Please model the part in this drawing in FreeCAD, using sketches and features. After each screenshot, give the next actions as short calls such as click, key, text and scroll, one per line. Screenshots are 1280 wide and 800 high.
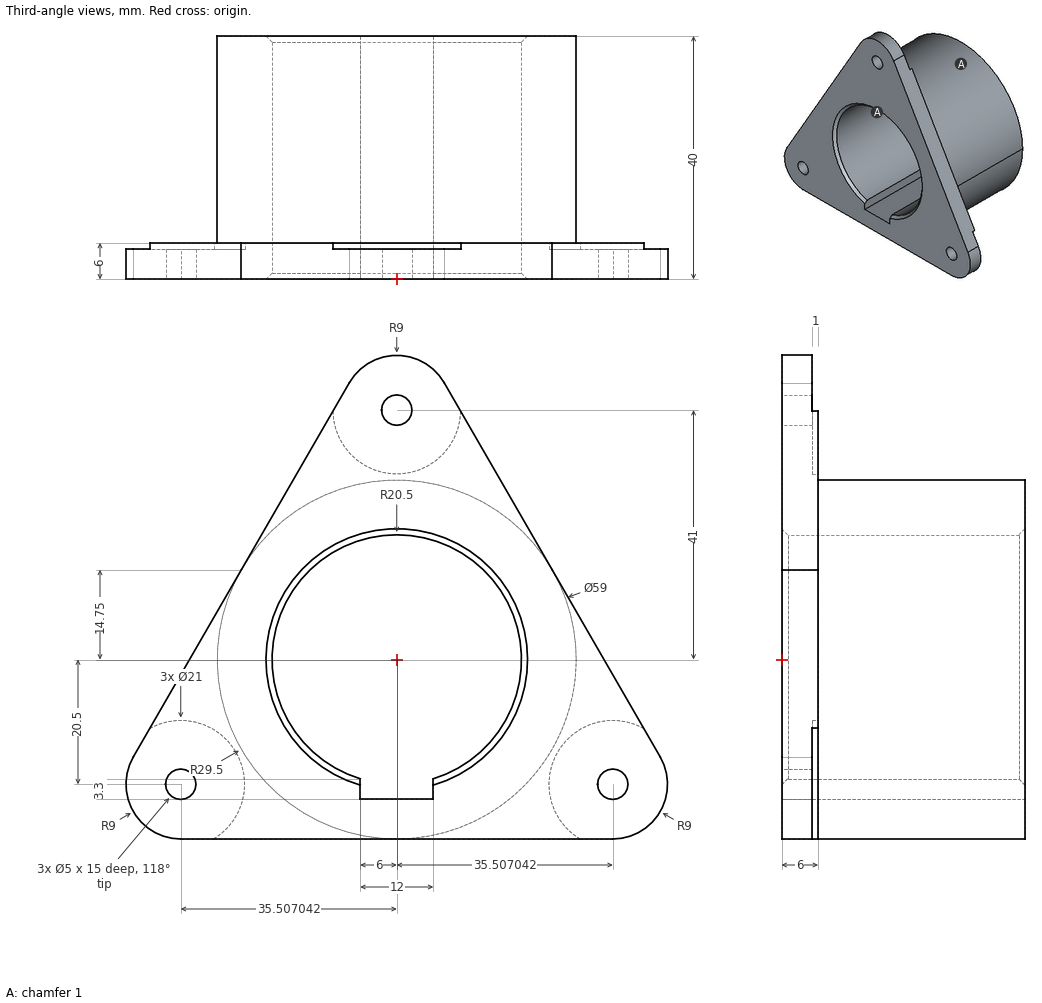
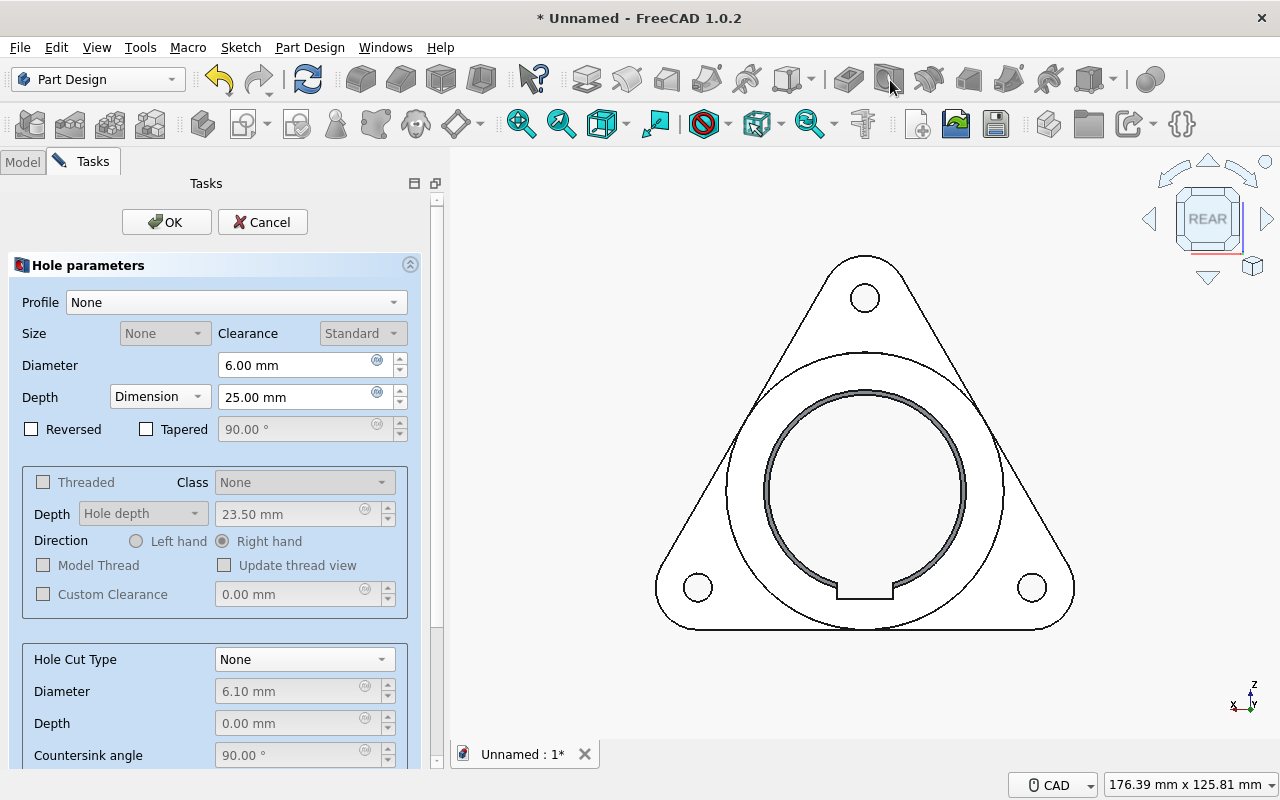
triple_click(305, 365)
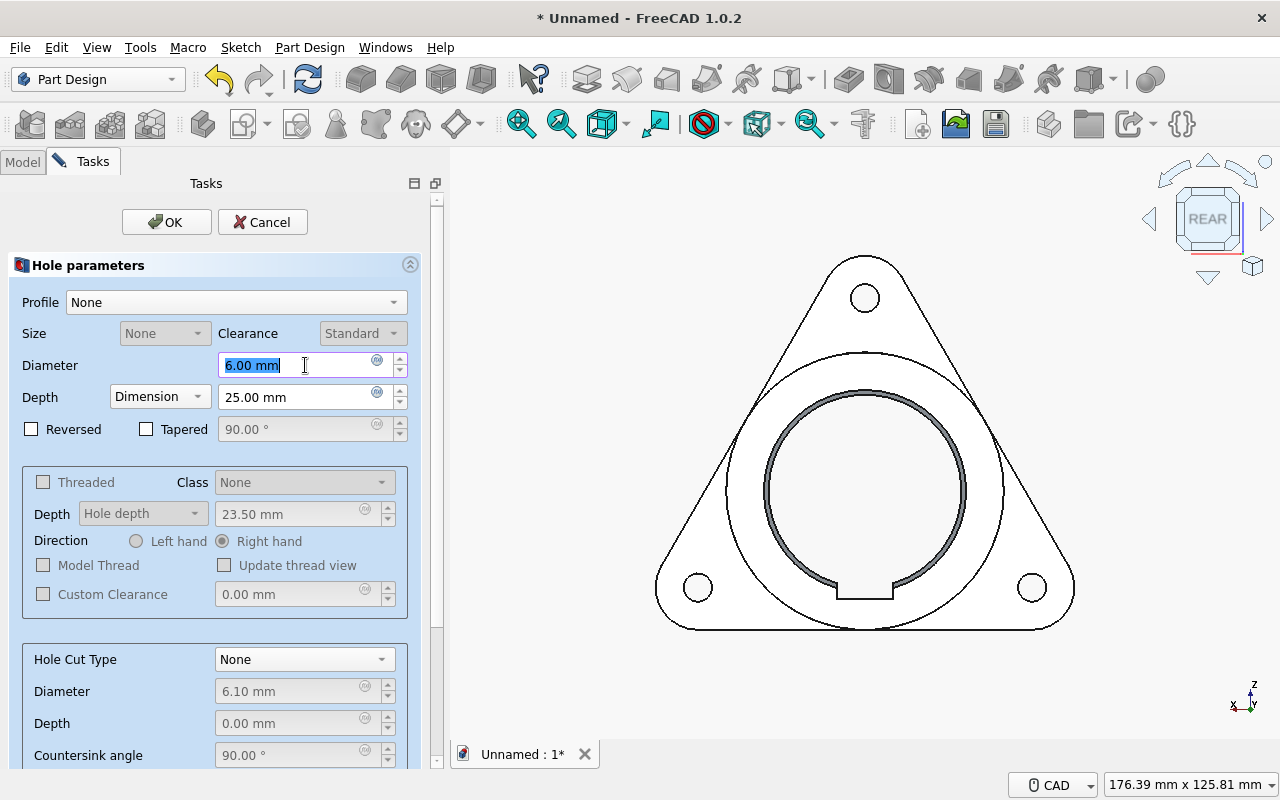
text(5)
key(Tab)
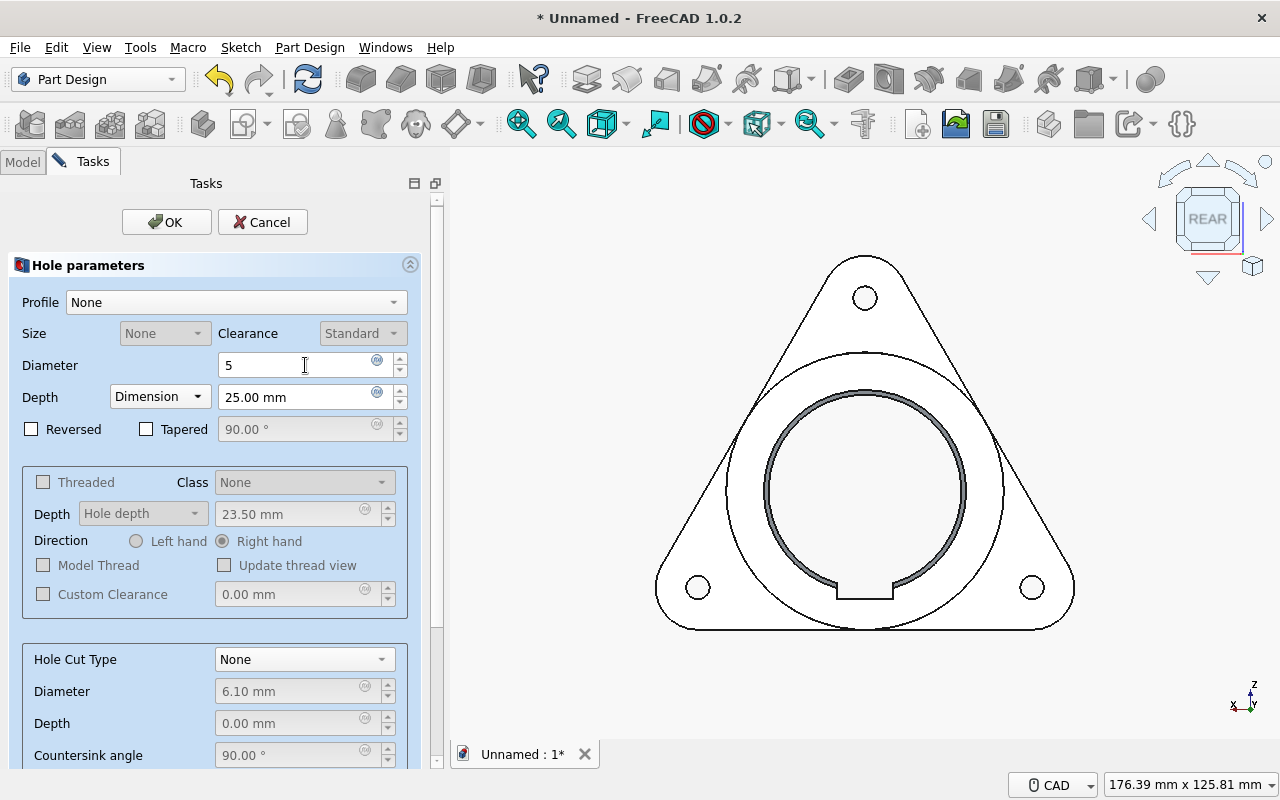
triple_click(305, 397)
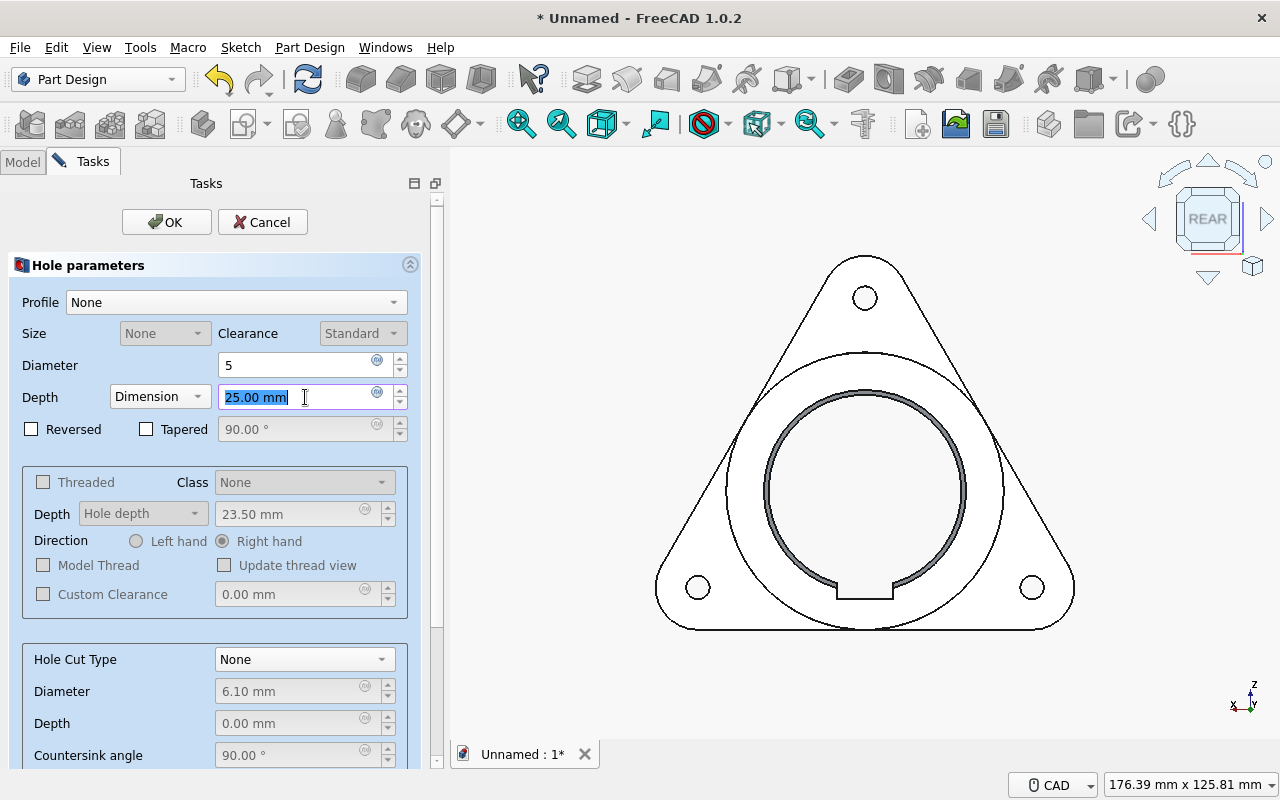
text(15)
key(Tab)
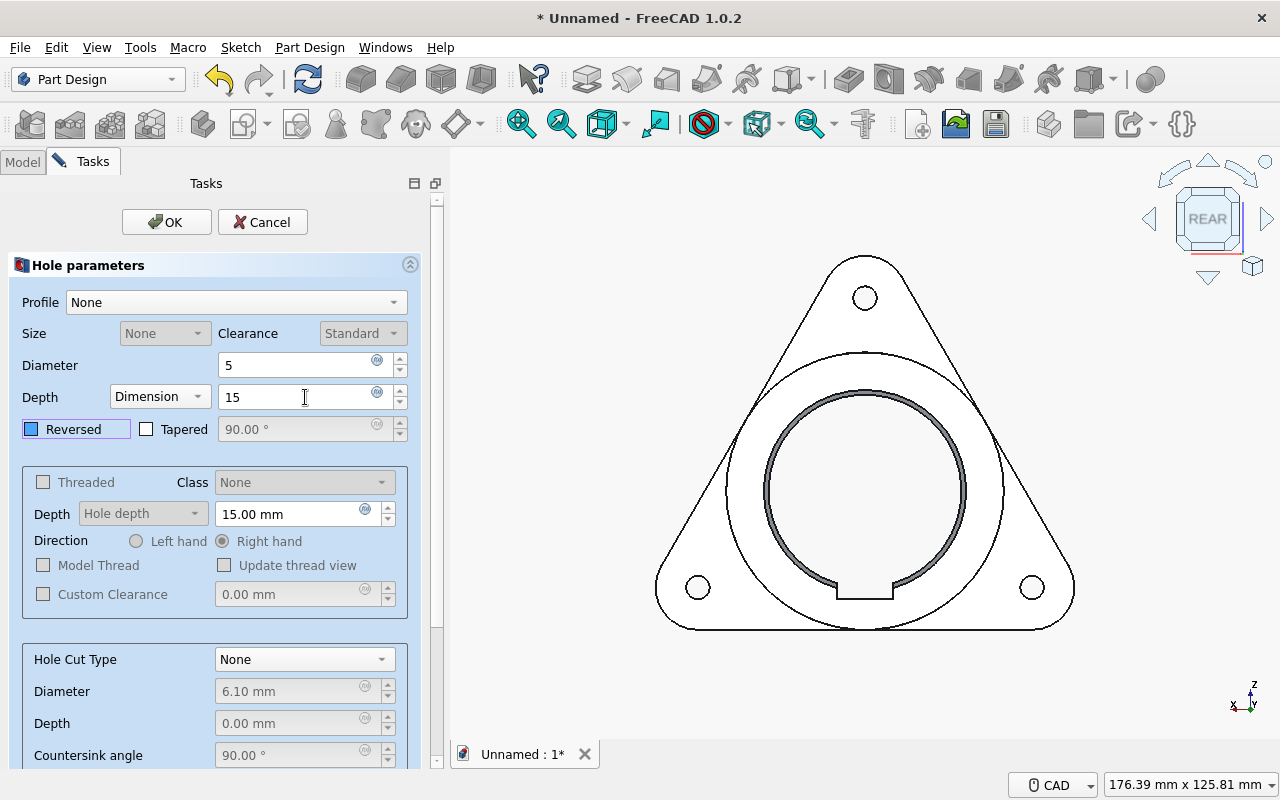
click(167, 222)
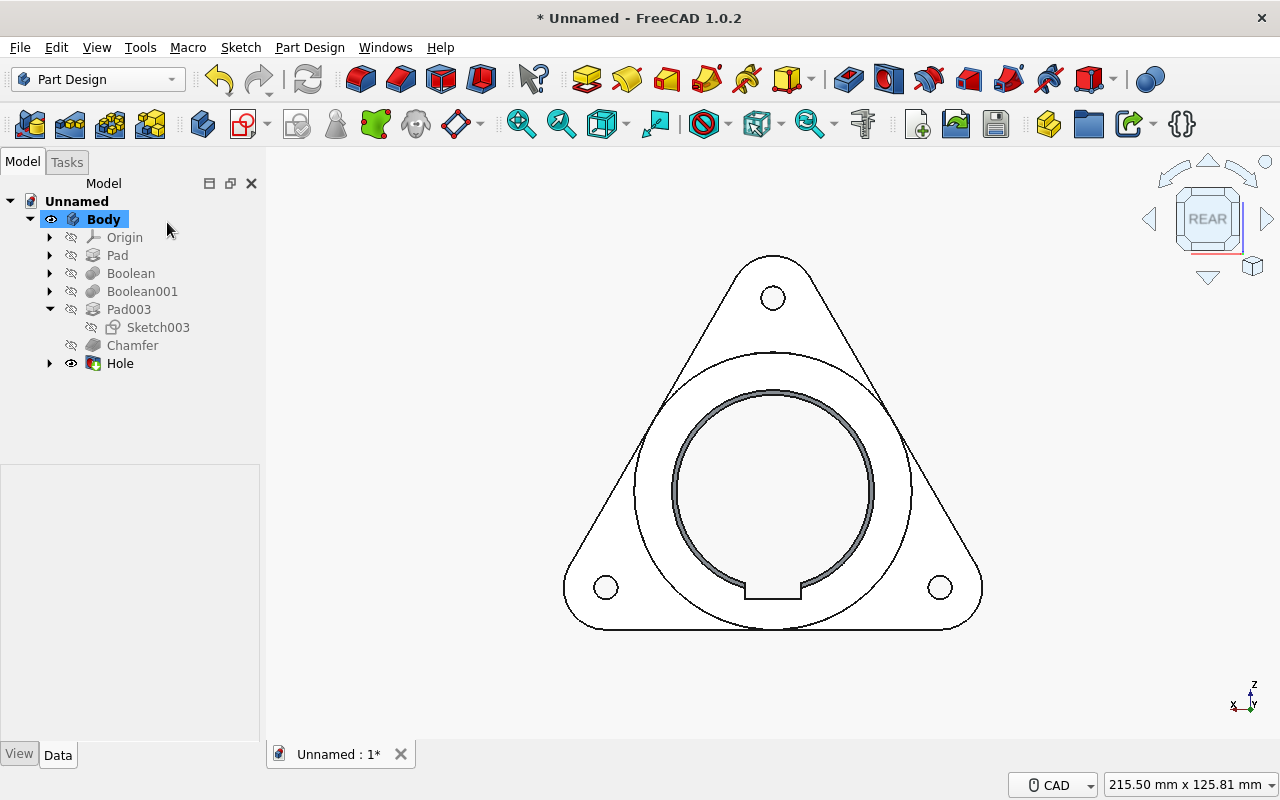
click(739, 314)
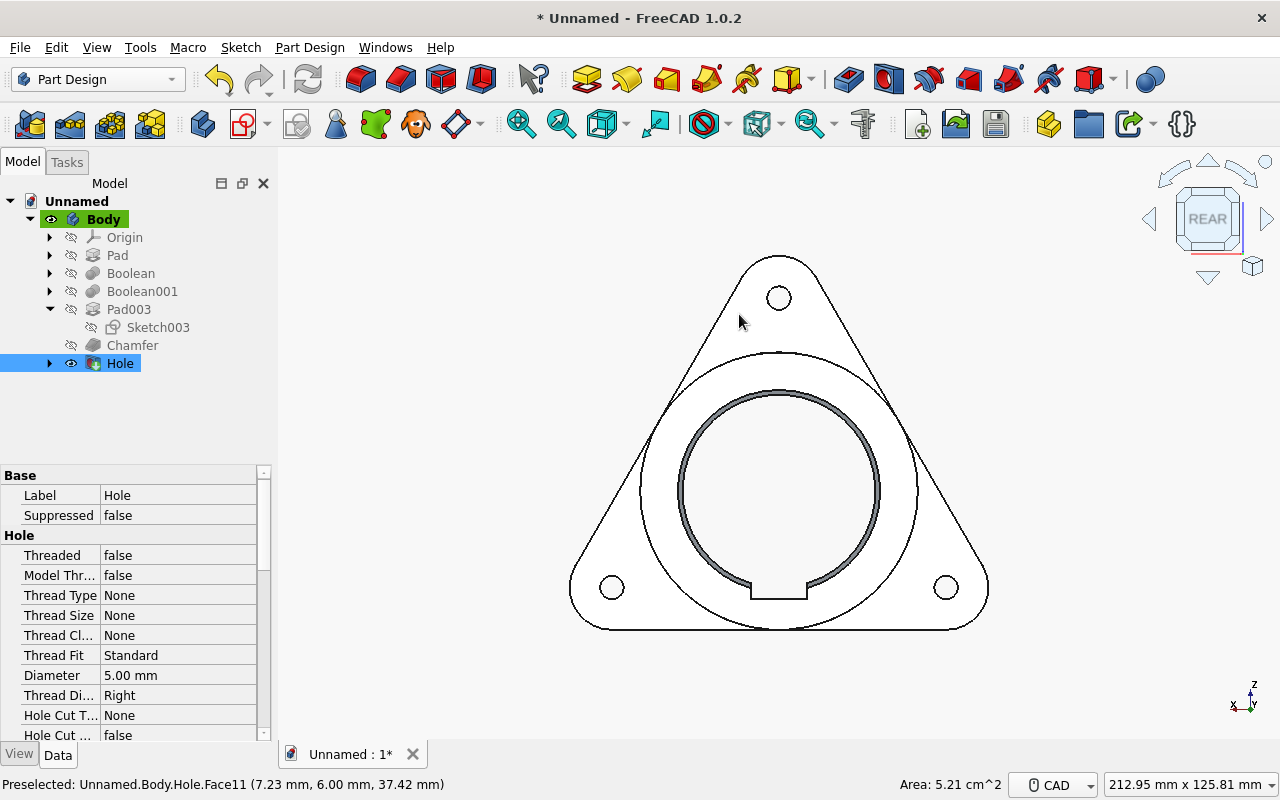
click(244, 124)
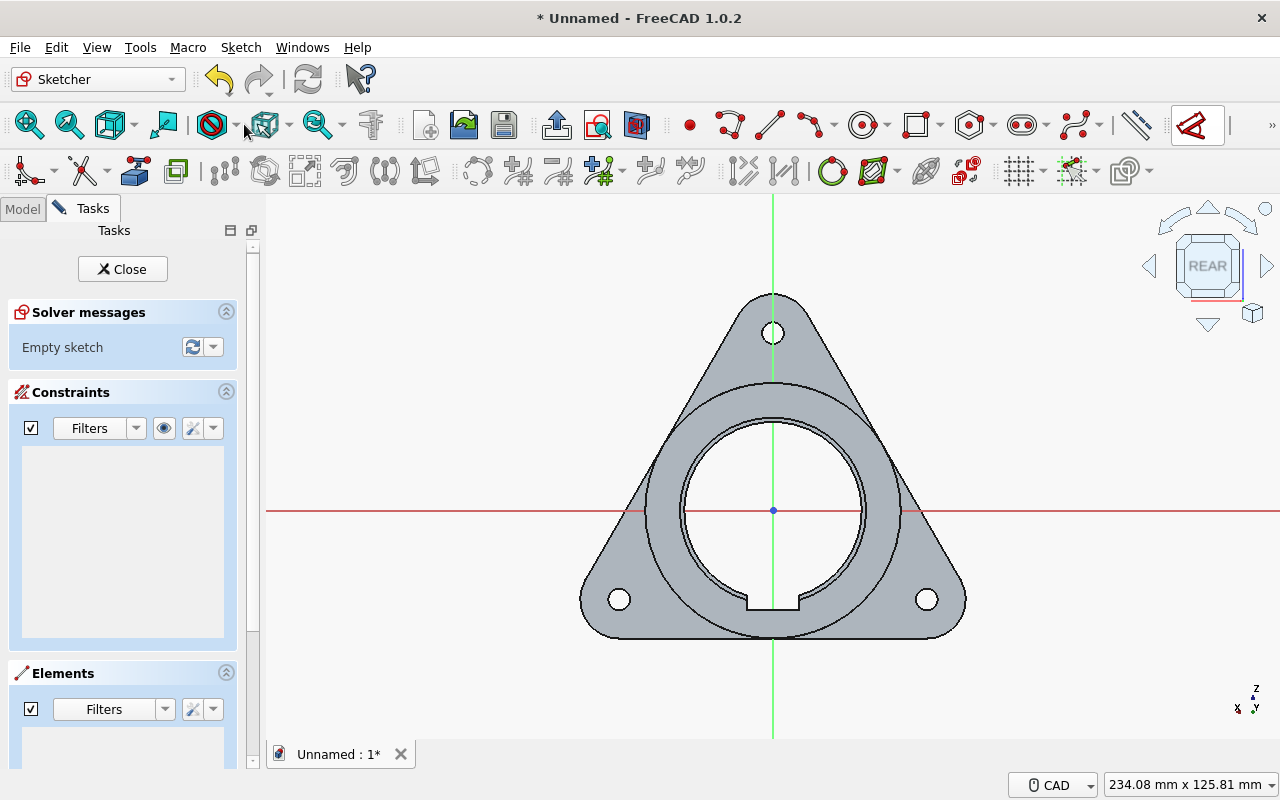
click(864, 126)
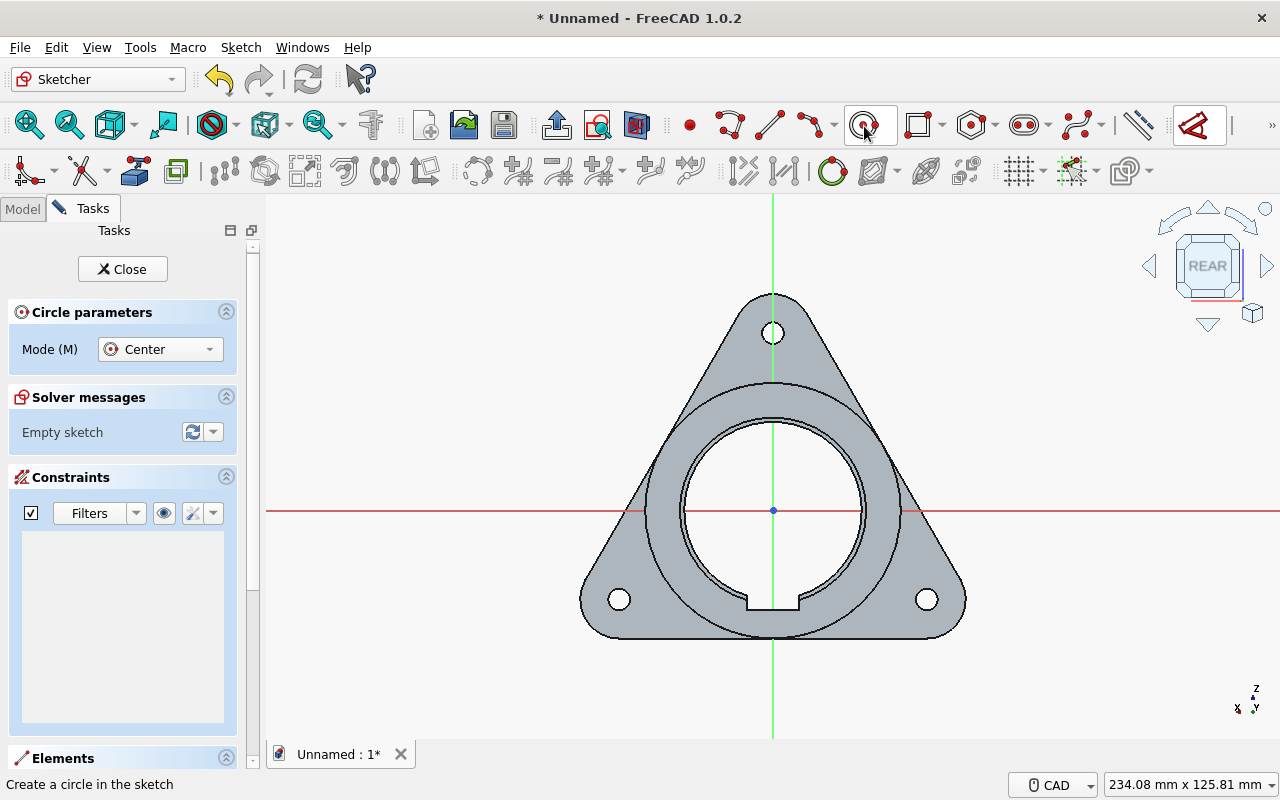
click(927, 600)
click(959, 567)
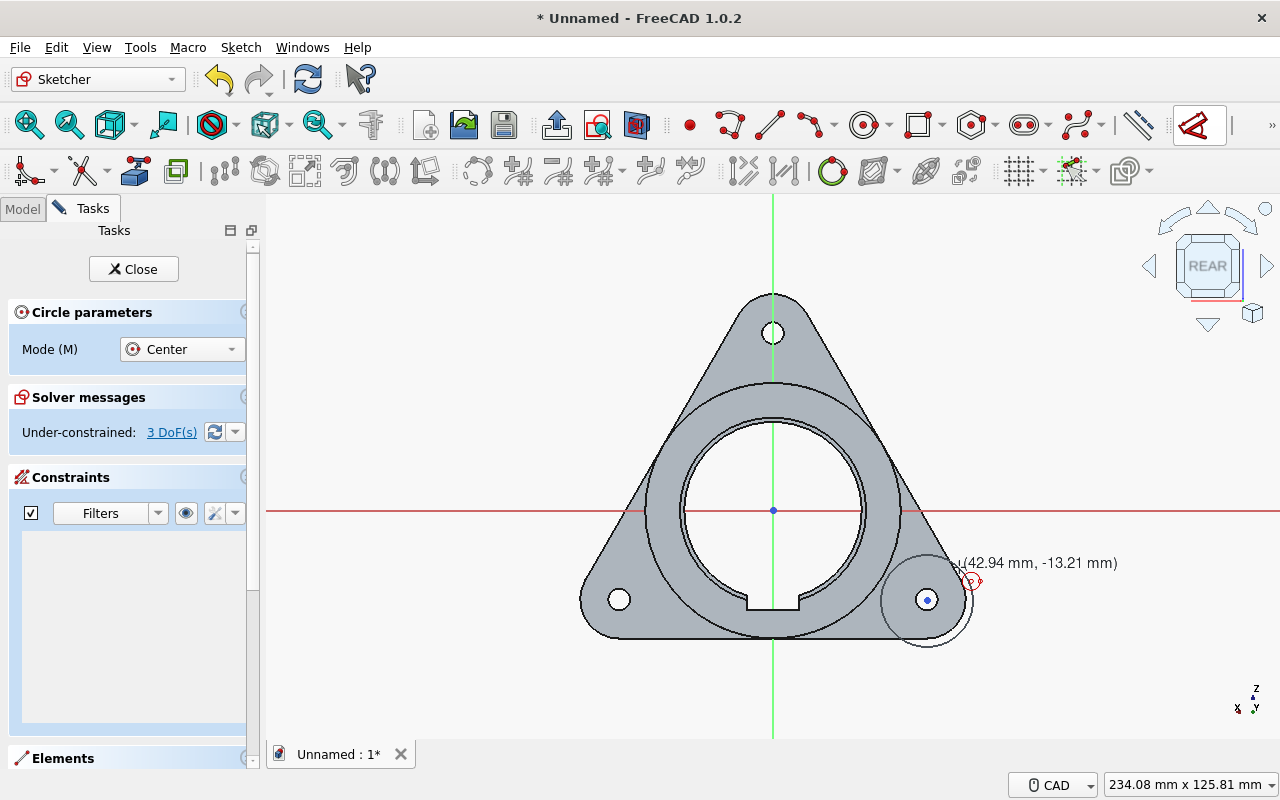
click(619, 600)
click(651, 567)